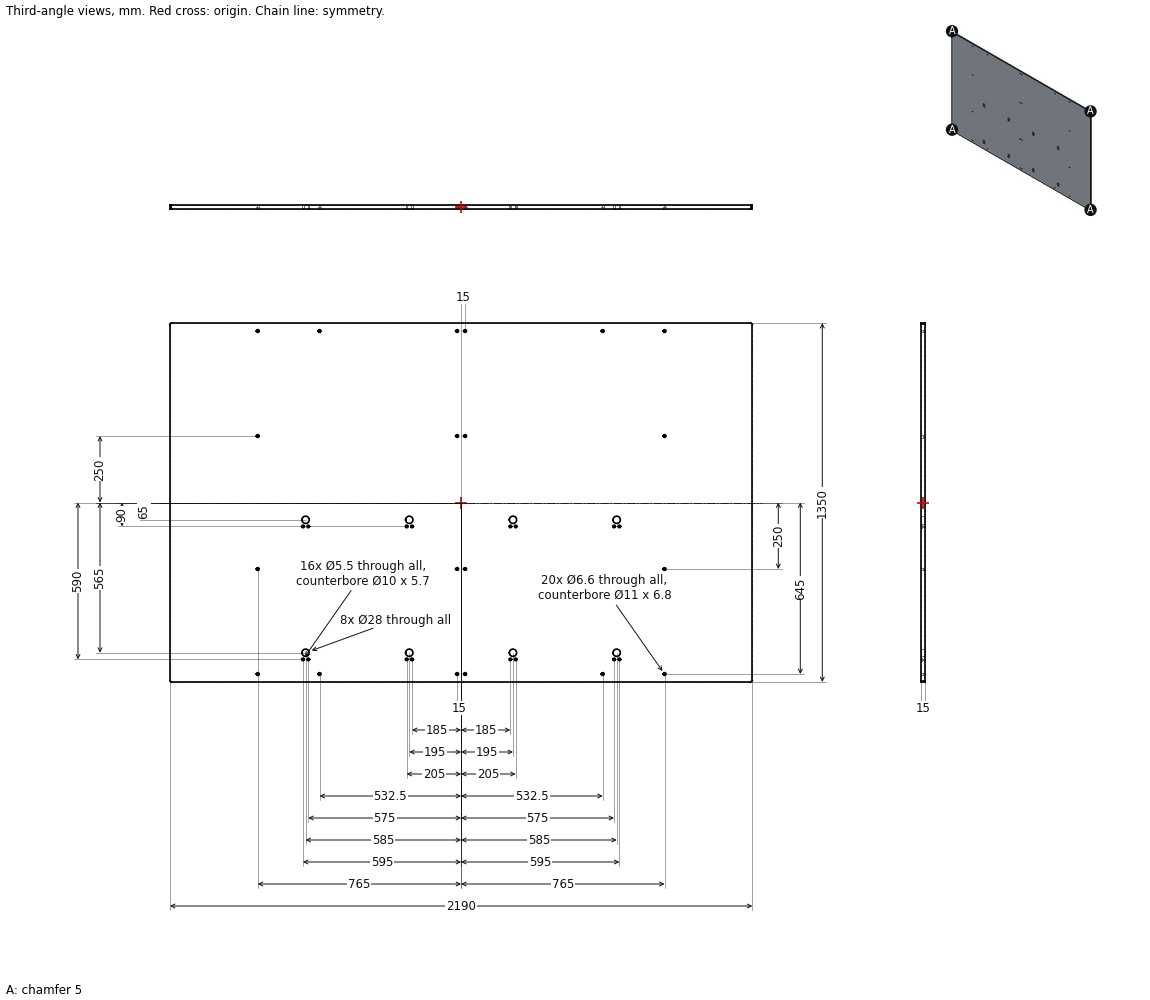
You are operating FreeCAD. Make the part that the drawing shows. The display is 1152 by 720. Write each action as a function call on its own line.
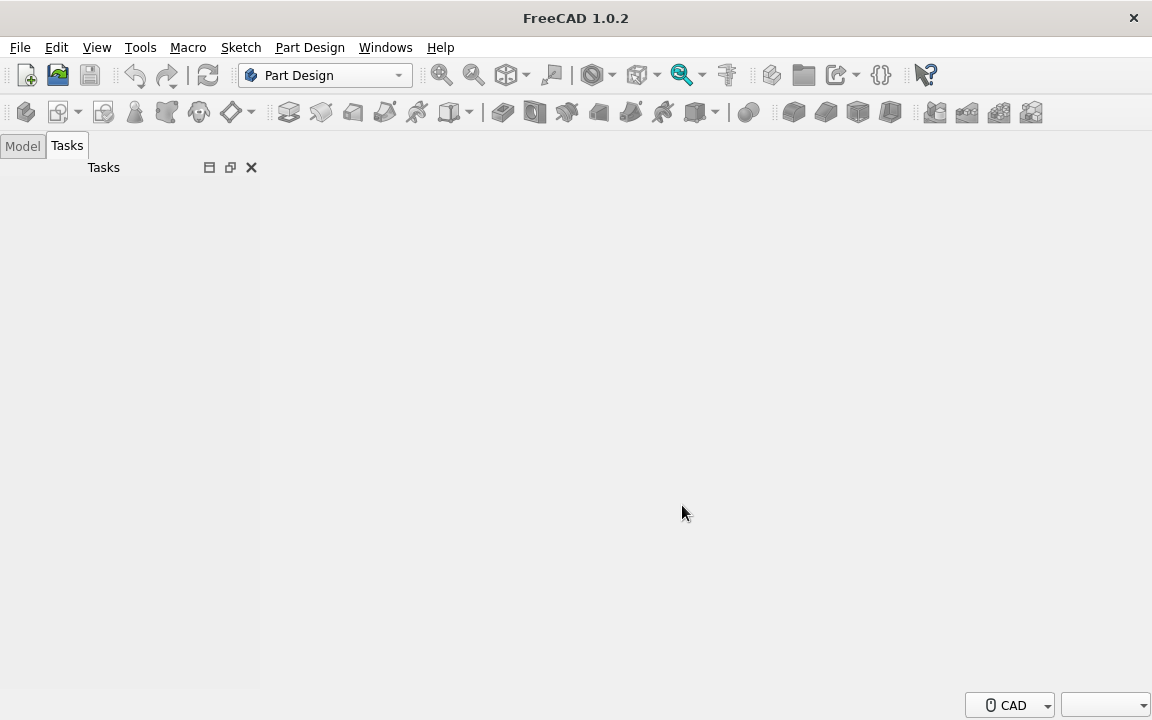
key(ctrl+n)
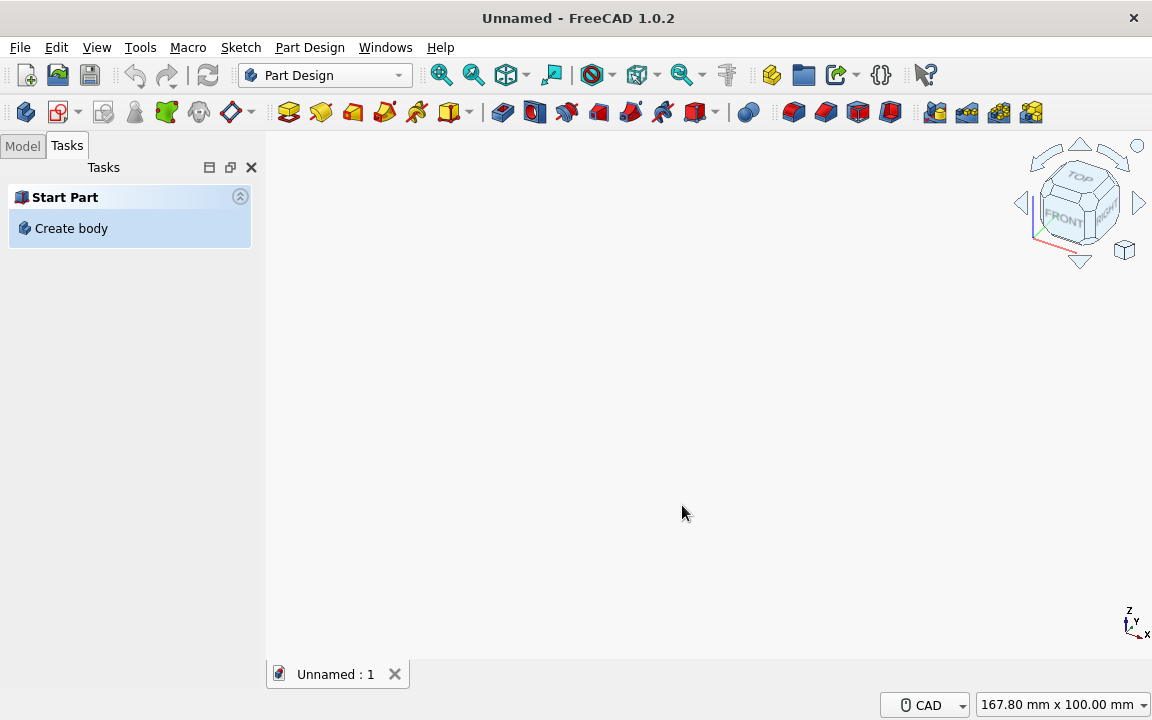
click(58, 112)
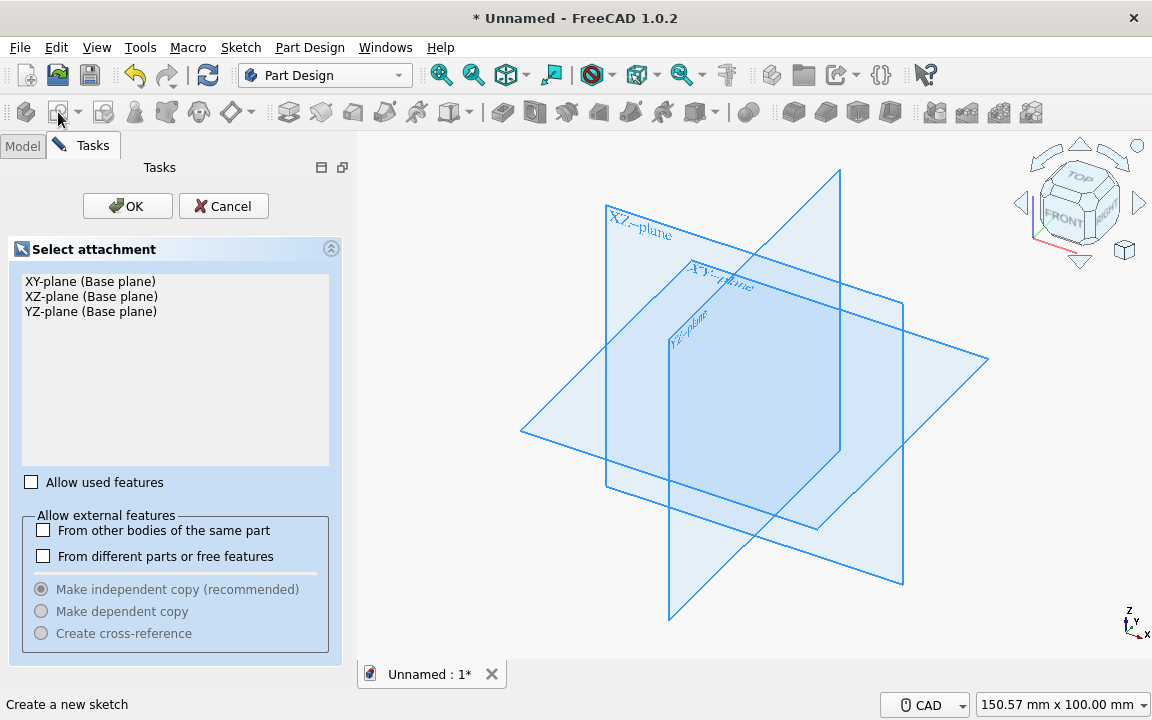
click(82, 296)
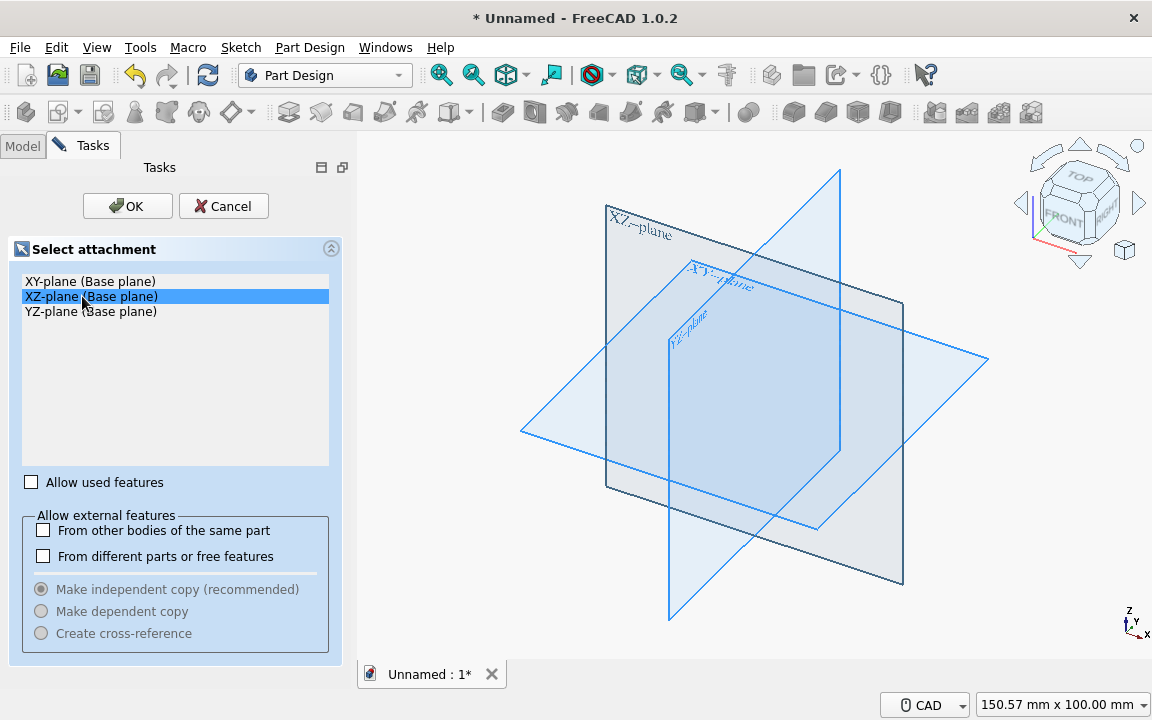
click(128, 206)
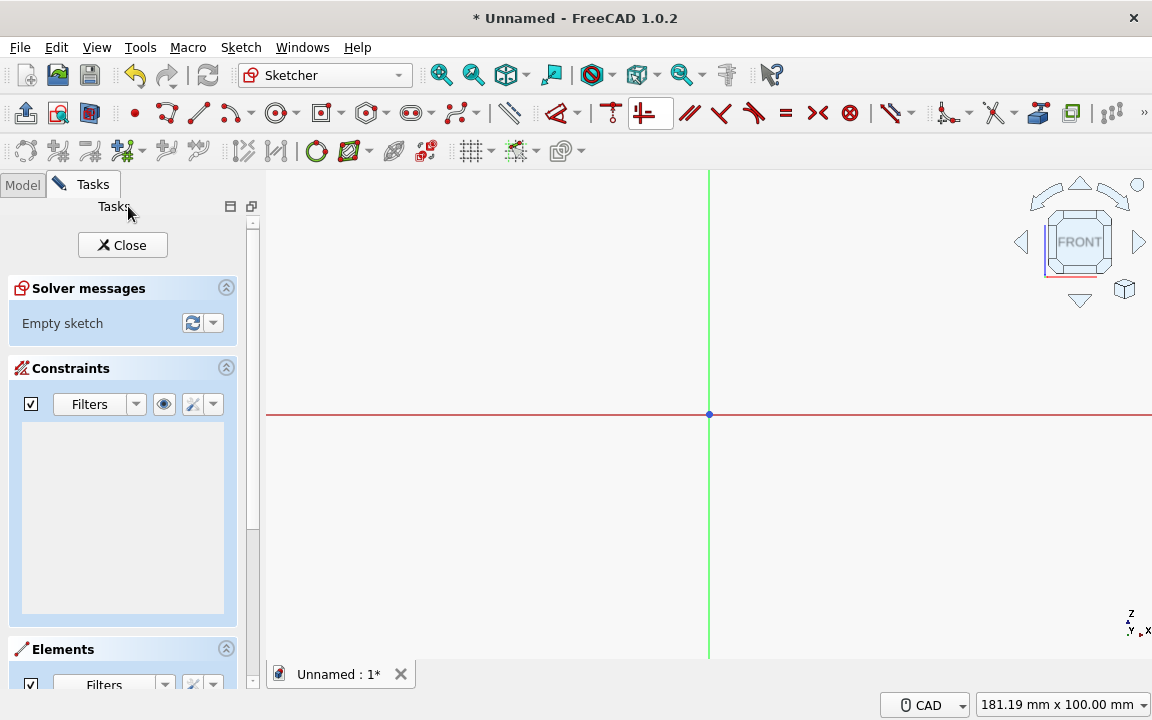
scroll(637, 414, down, 15)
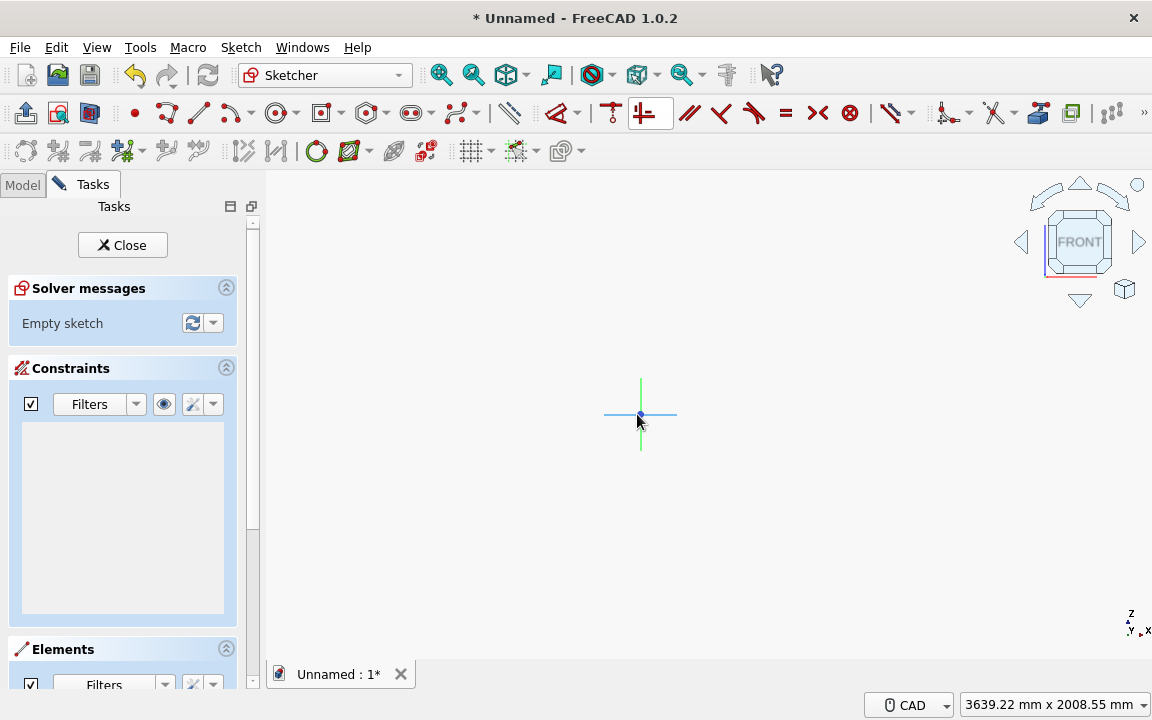
click(322, 114)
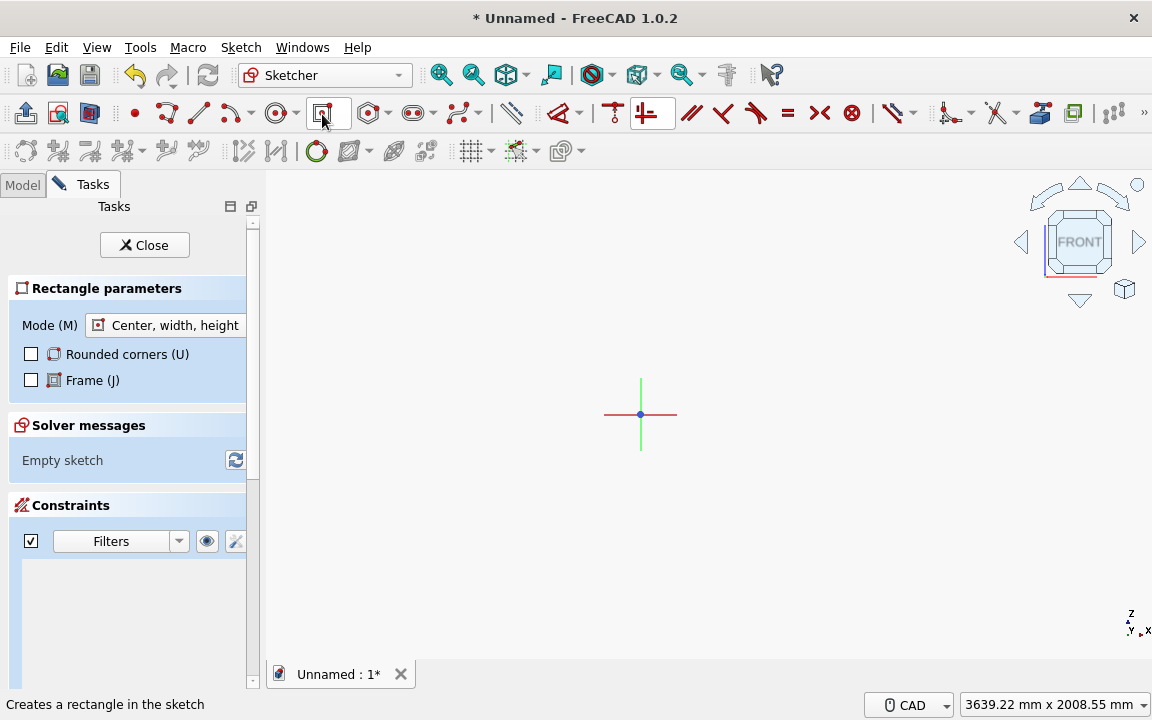
click(641, 414)
move(908, 250)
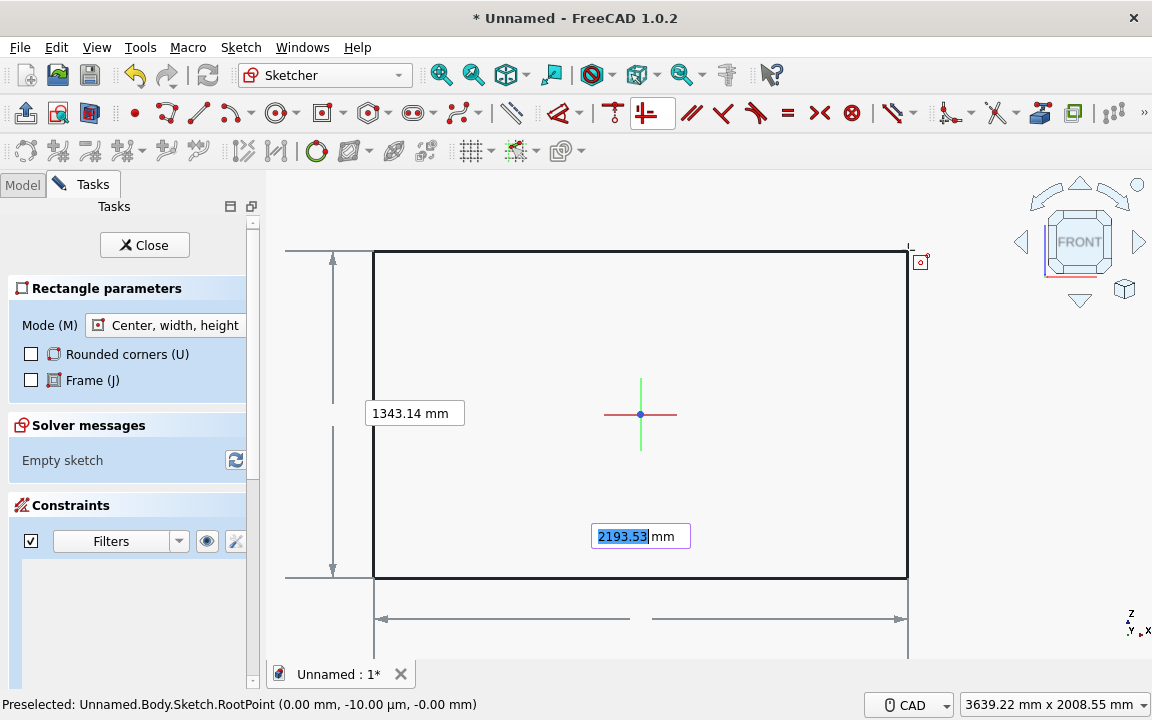
text(2190)
key(Tab)
text(1350)
key(Return)
key(Escape)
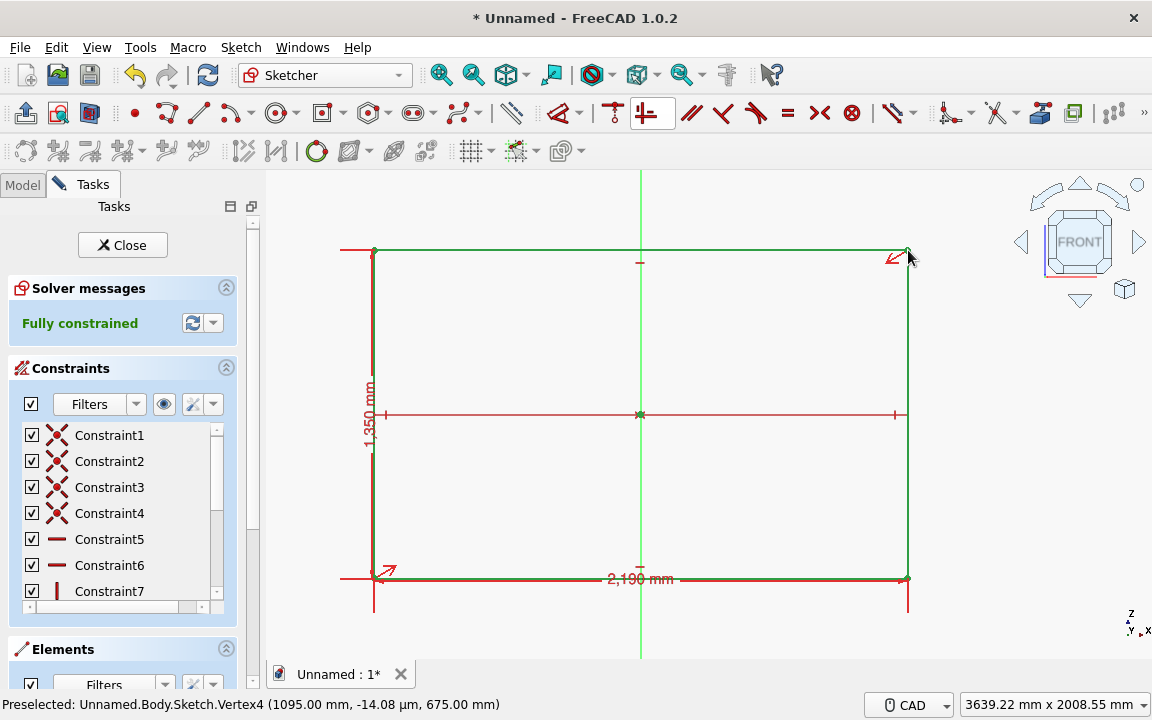
click(123, 245)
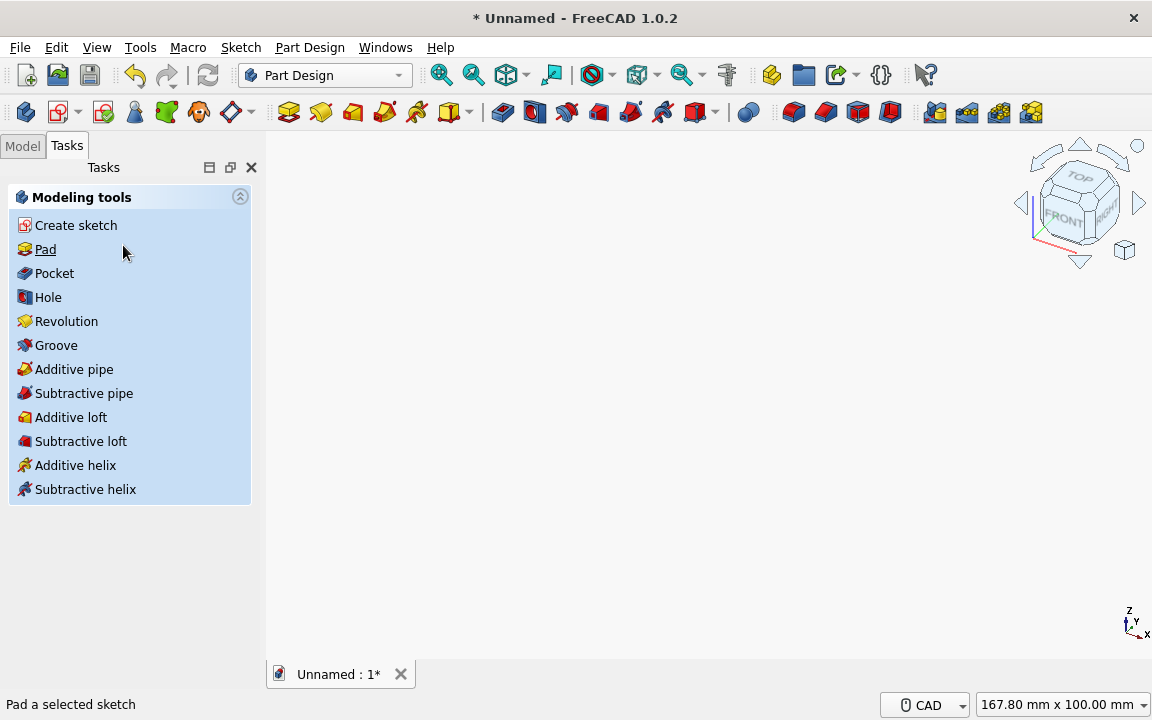
click(290, 112)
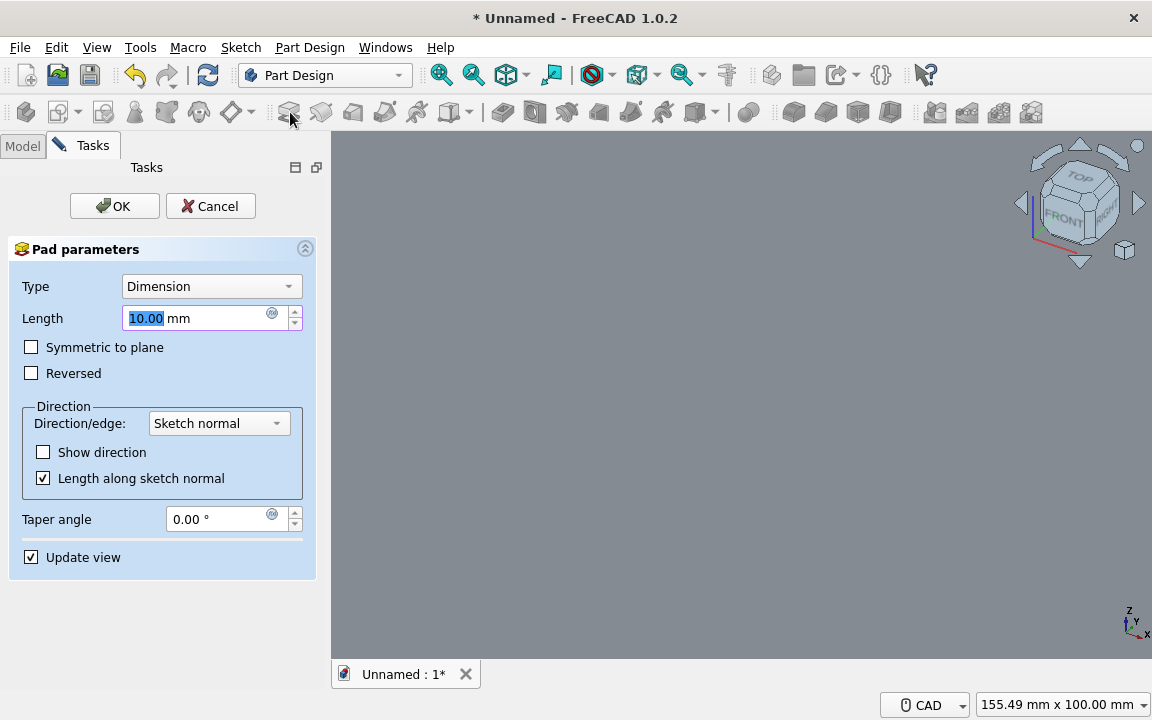
text(15)
key(Tab)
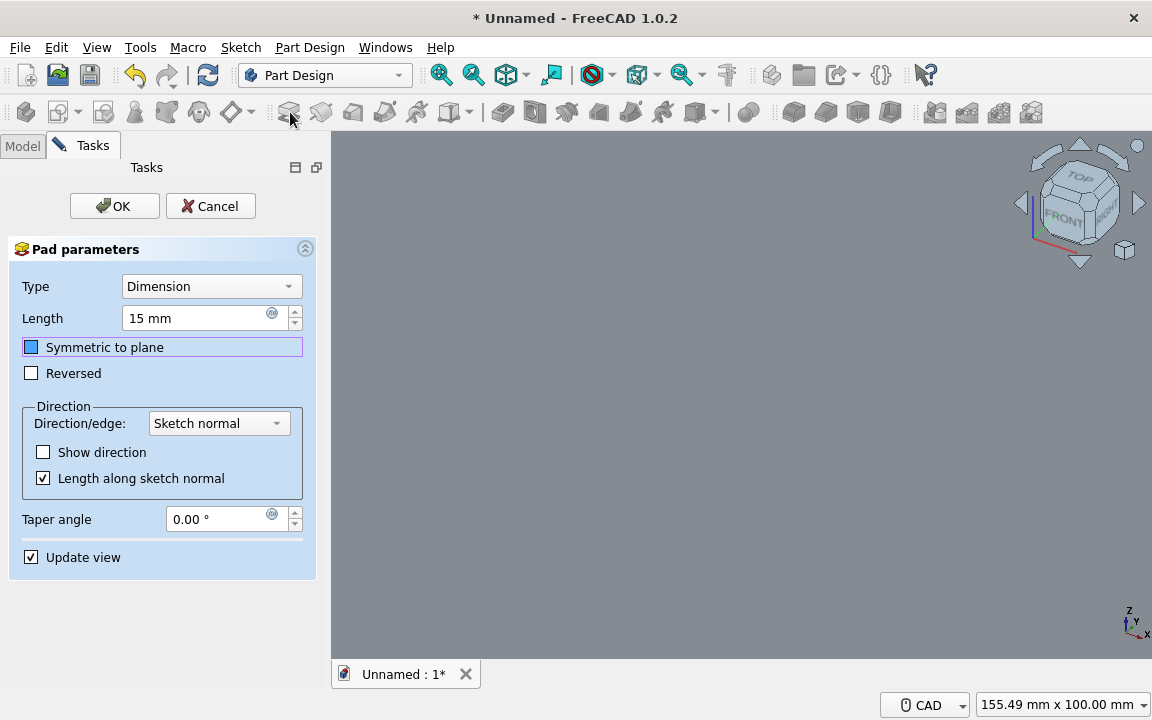
click(30, 347)